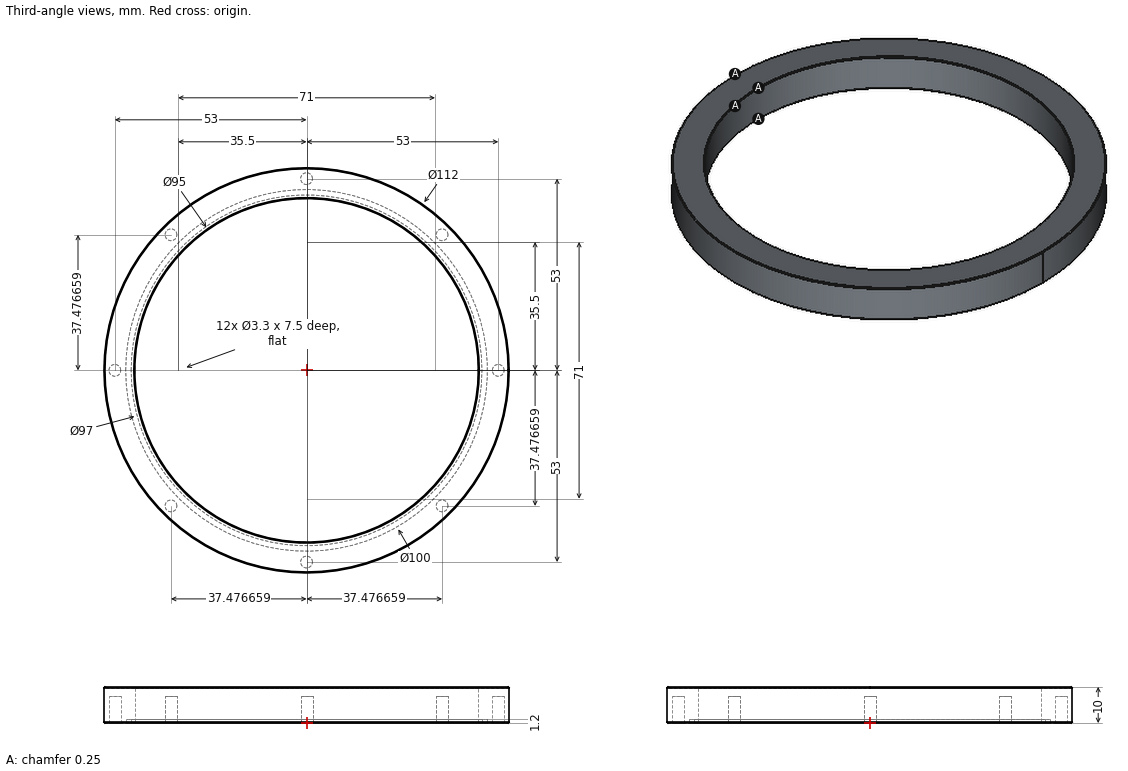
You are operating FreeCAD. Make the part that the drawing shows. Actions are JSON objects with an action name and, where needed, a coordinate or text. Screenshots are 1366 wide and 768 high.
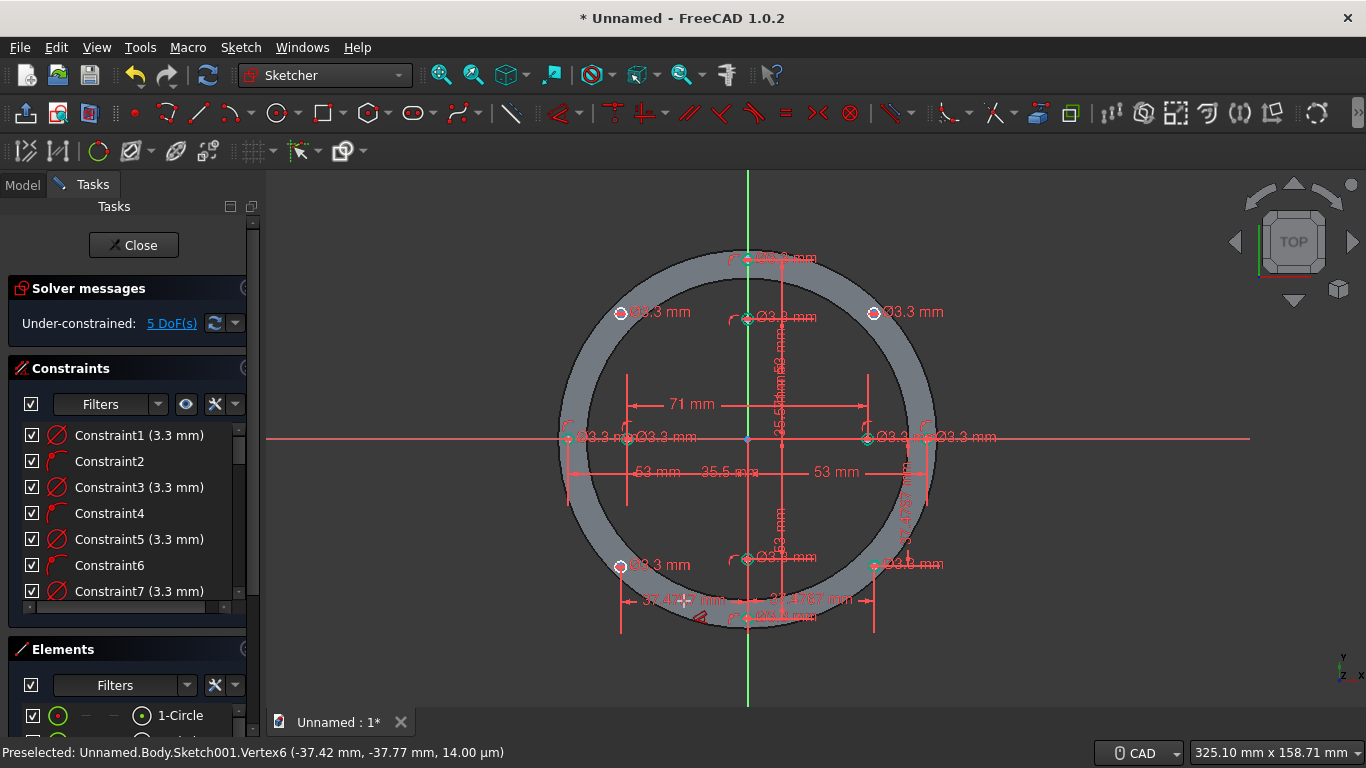
{"action": "left_click", "coordinate": [621, 567]}
{"action": "left_click", "coordinate": [587, 503]}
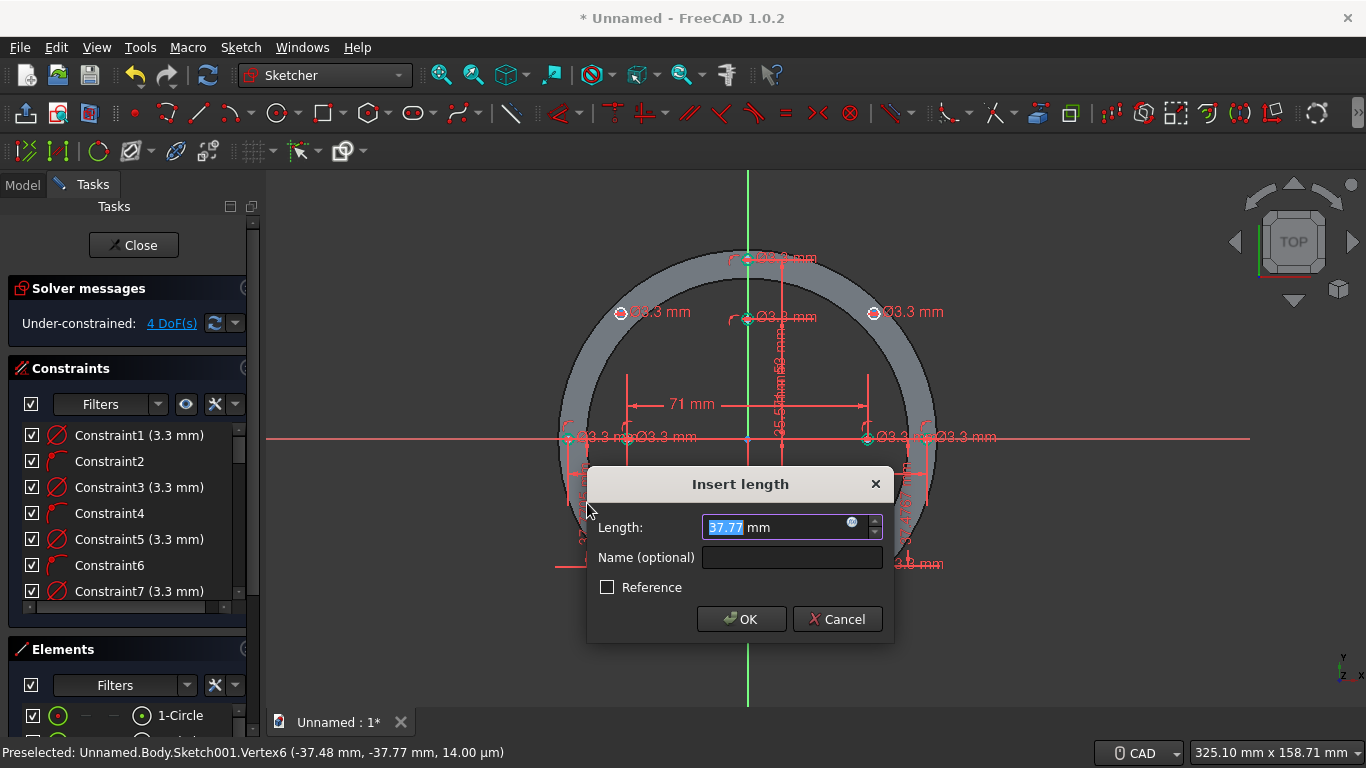
{"action": "type", "text": "37.476659"}
{"action": "key", "text": "Return"}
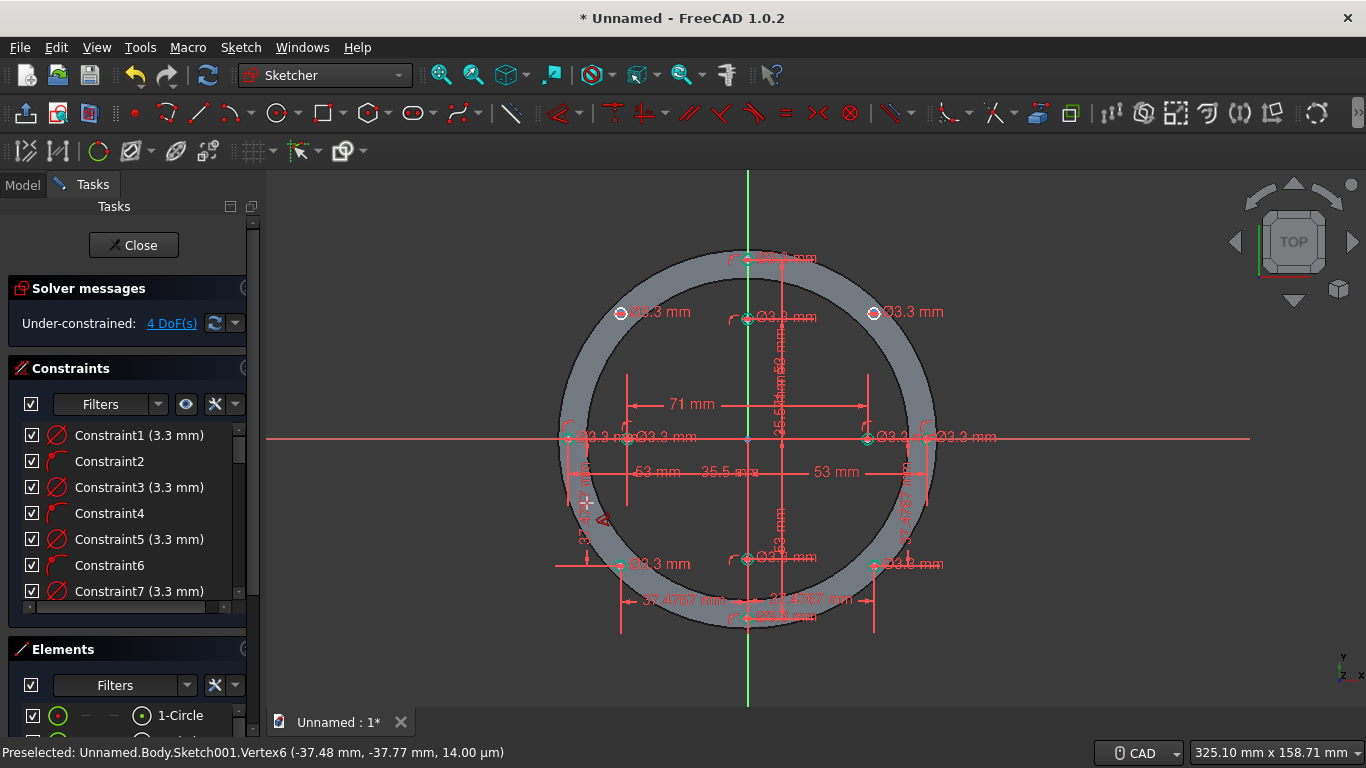
{"action": "left_click", "coordinate": [621, 314]}
{"action": "left_click", "coordinate": [684, 280]}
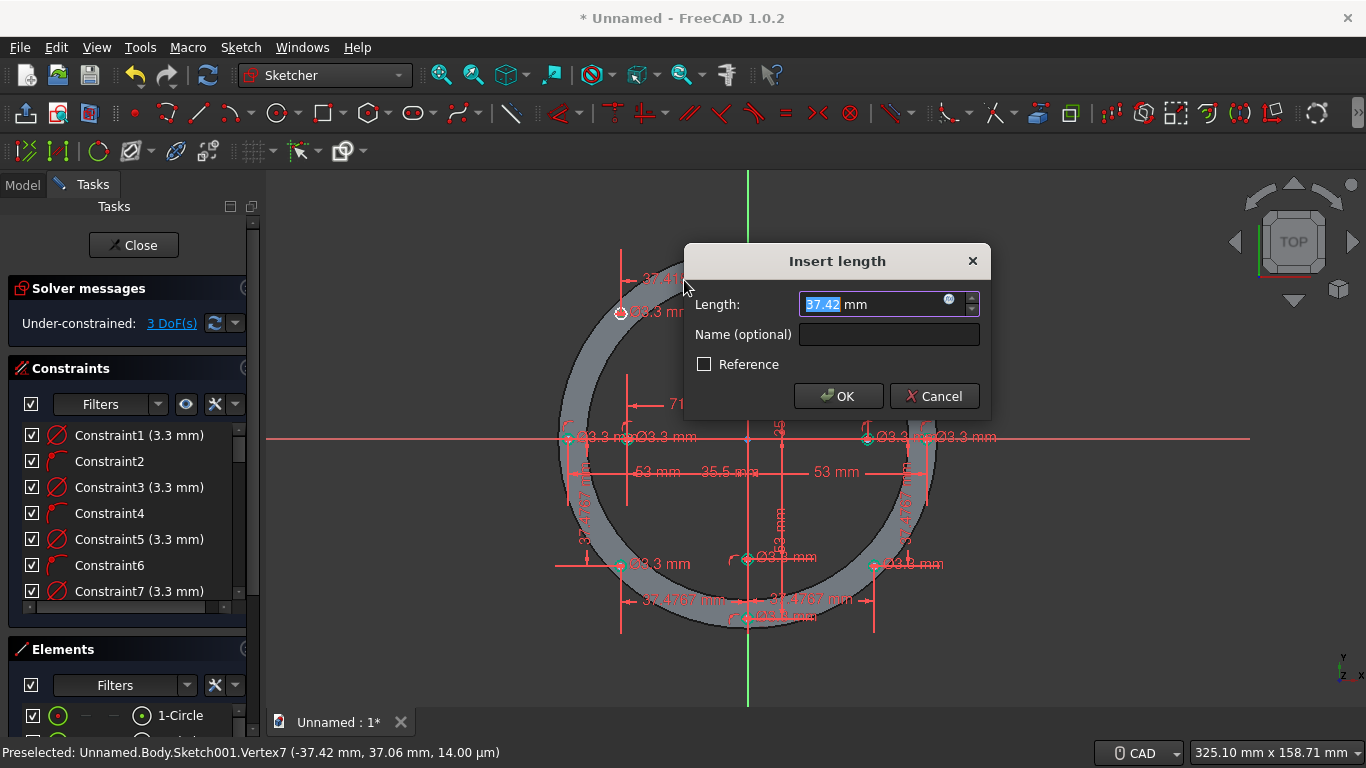
{"action": "type", "text": "37.476659"}
{"action": "key", "text": "Return"}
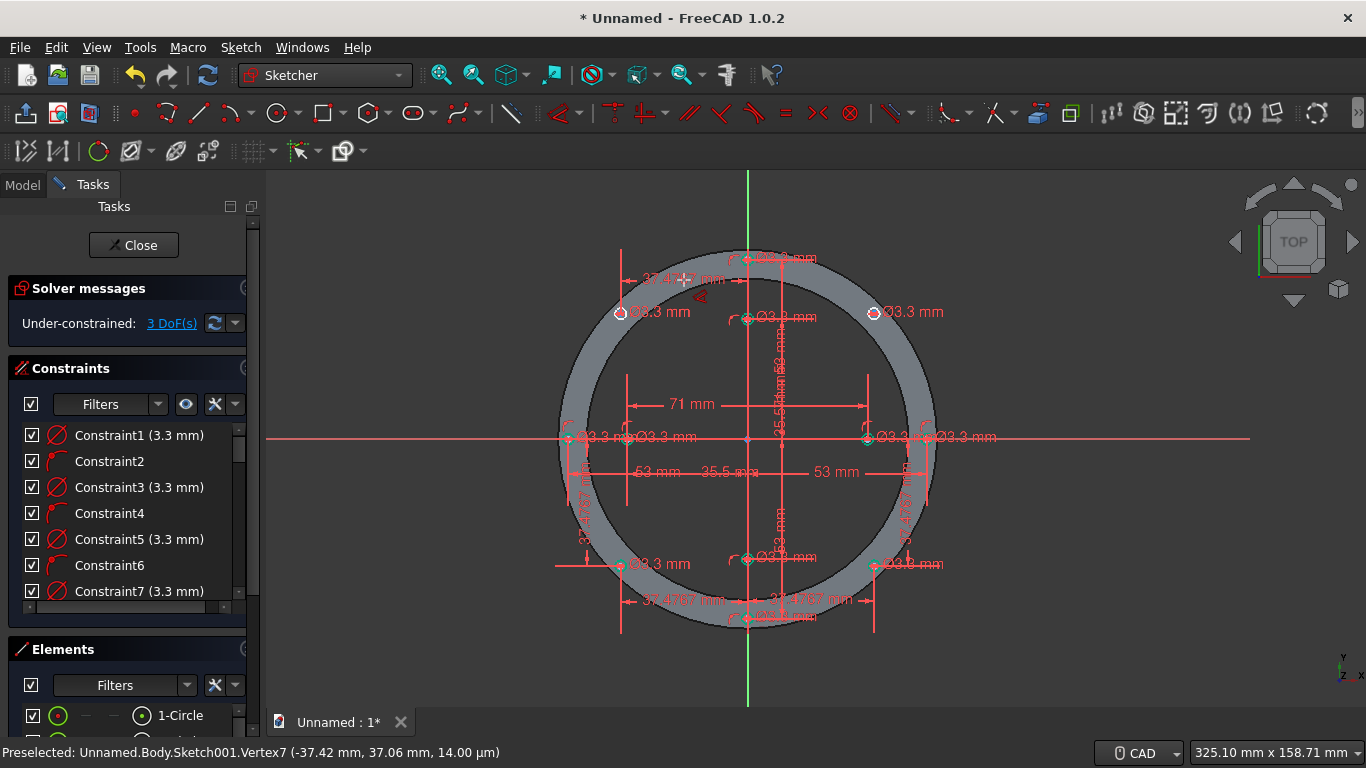
{"action": "left_click", "coordinate": [621, 314]}
{"action": "left_click", "coordinate": [587, 376]}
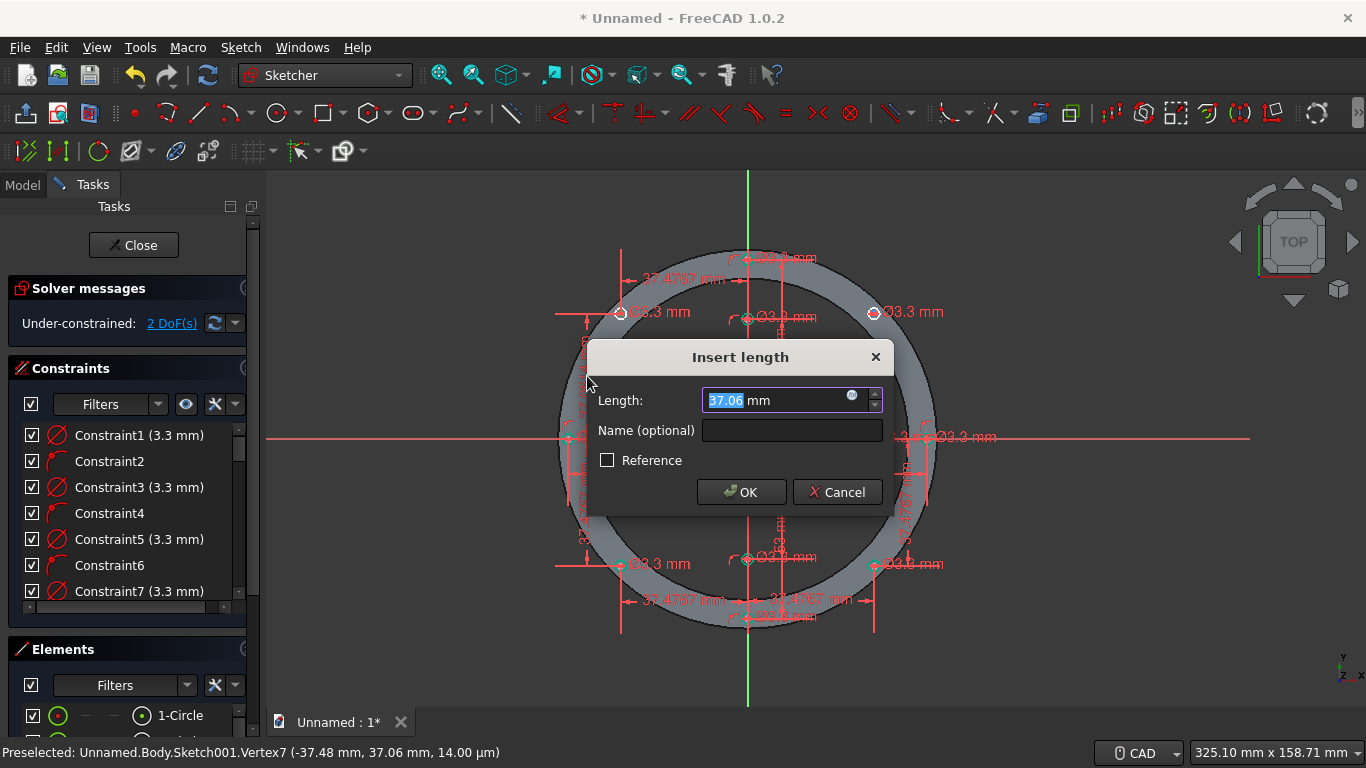
{"action": "type", "text": "37.476659"}
{"action": "key", "text": "Return"}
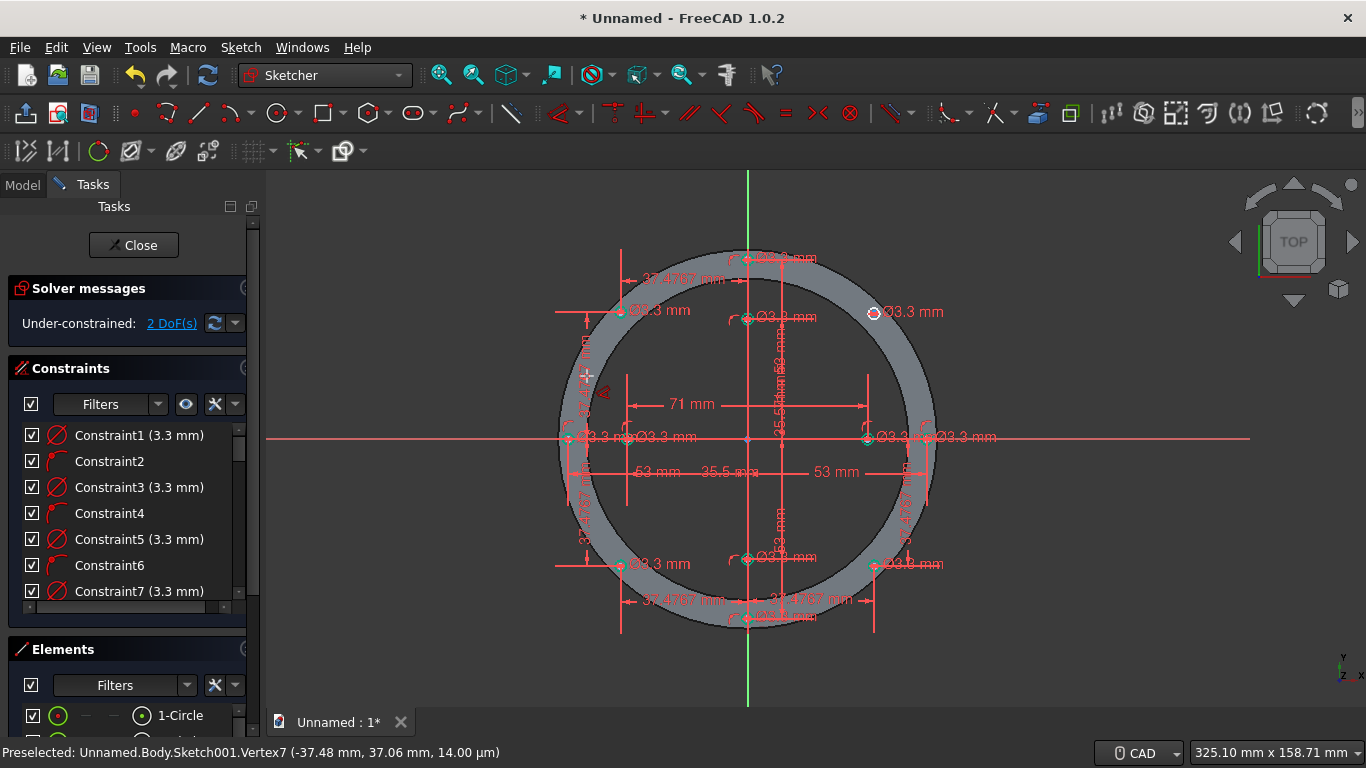
{"action": "left_click", "coordinate": [874, 314]}
{"action": "left_click", "coordinate": [811, 280]}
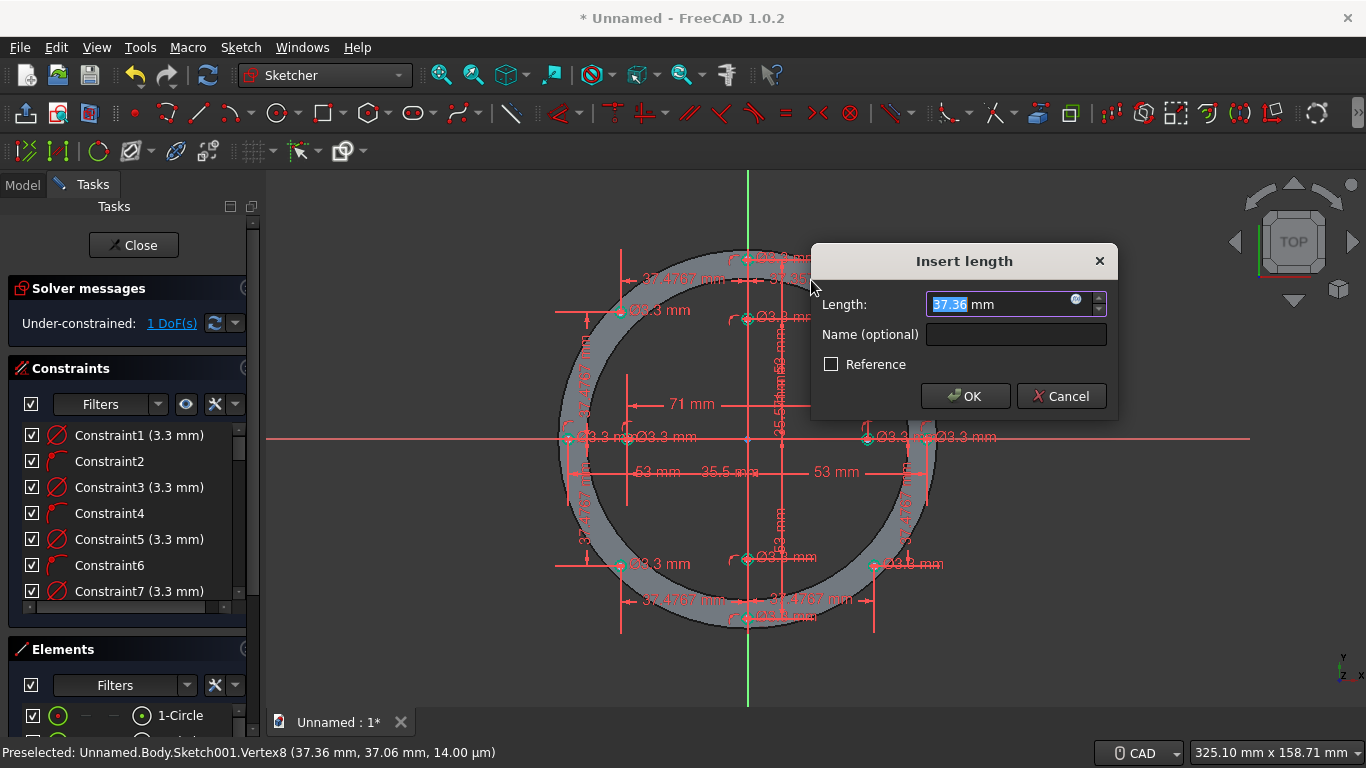
{"action": "type", "text": "37.476659"}
{"action": "key", "text": "Return"}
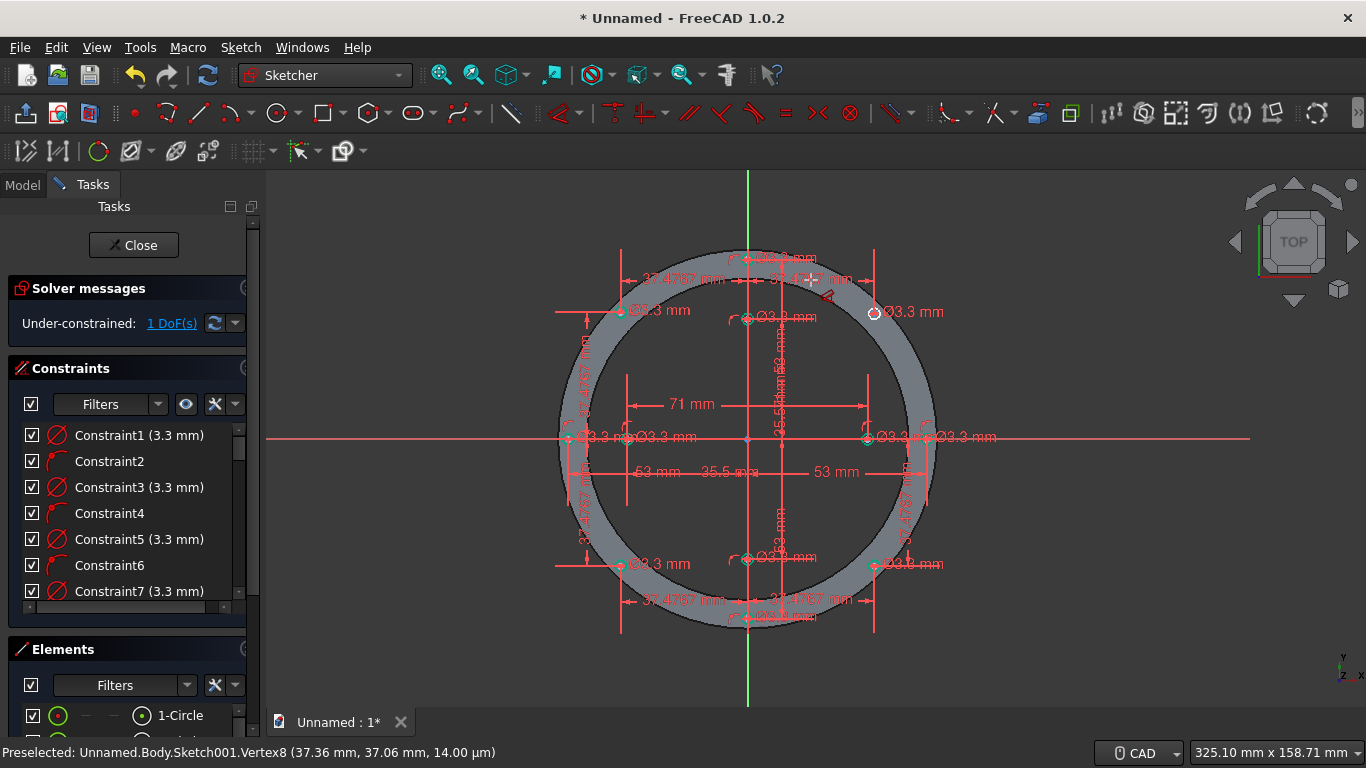
{"action": "left_click", "coordinate": [874, 314]}
{"action": "left_click", "coordinate": [908, 376]}